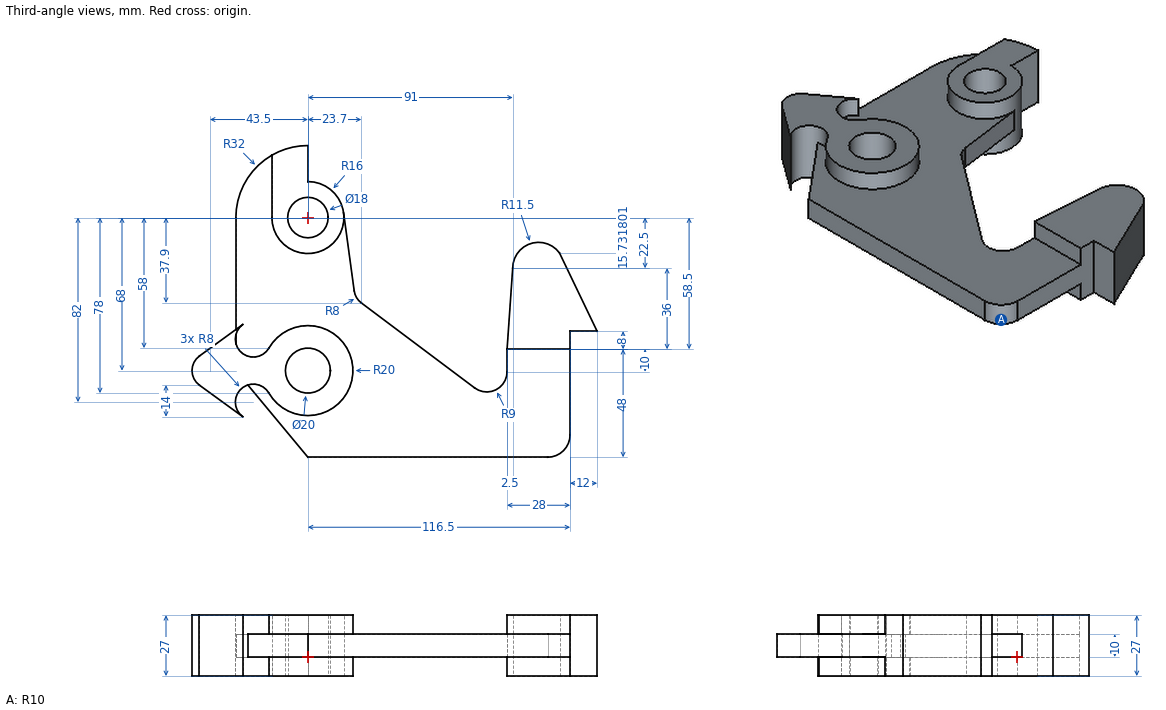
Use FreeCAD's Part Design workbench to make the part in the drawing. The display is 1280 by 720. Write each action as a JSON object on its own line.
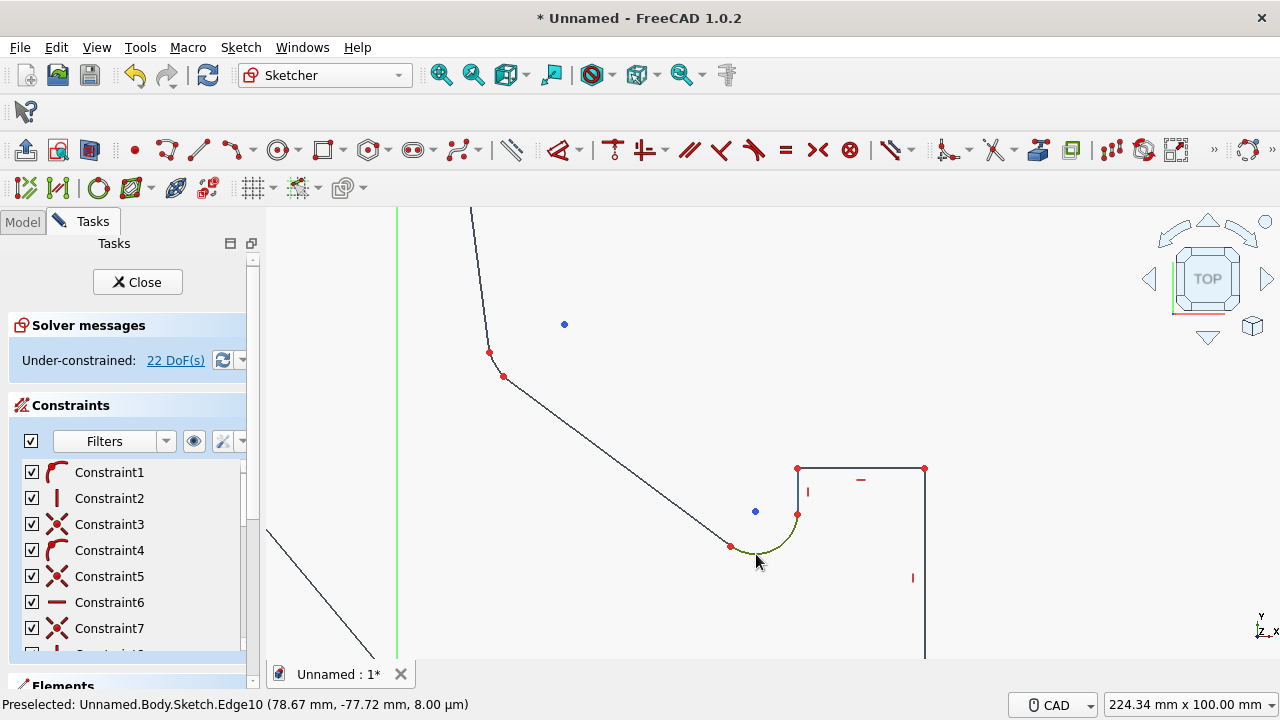
{"action": "left_click", "coordinate": [754, 150]}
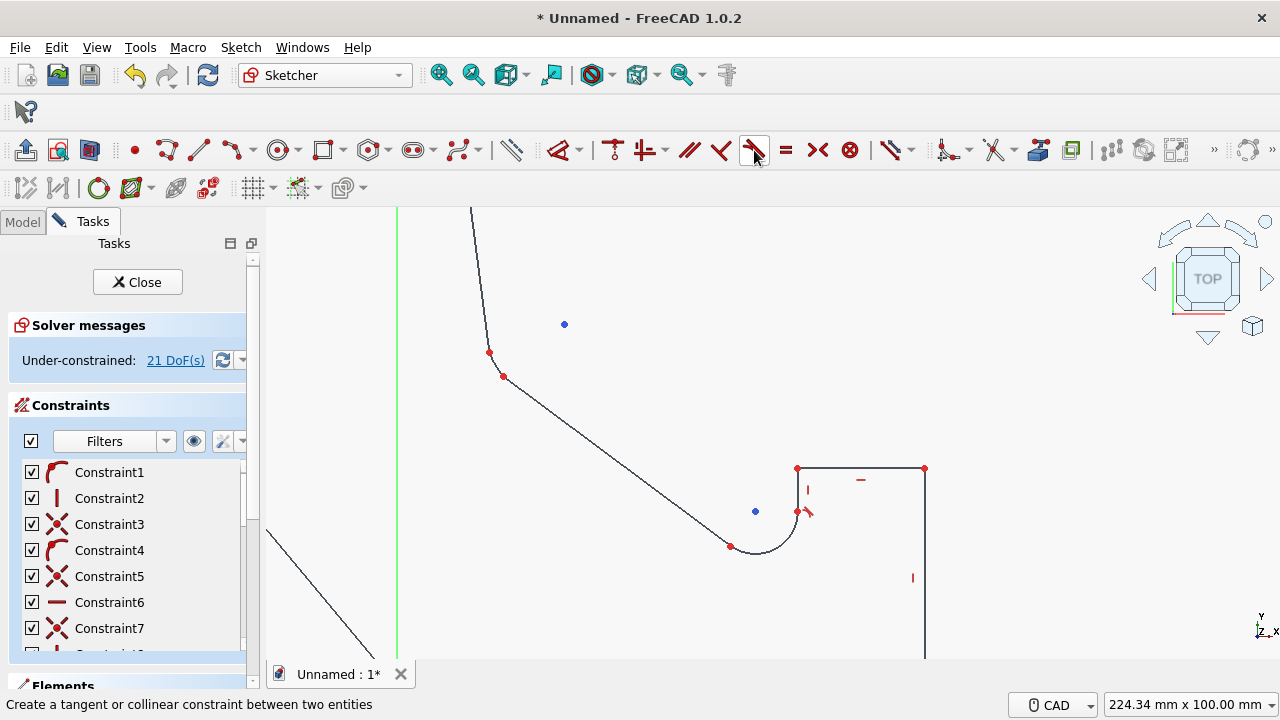
{"action": "left_click", "coordinate": [663, 495]}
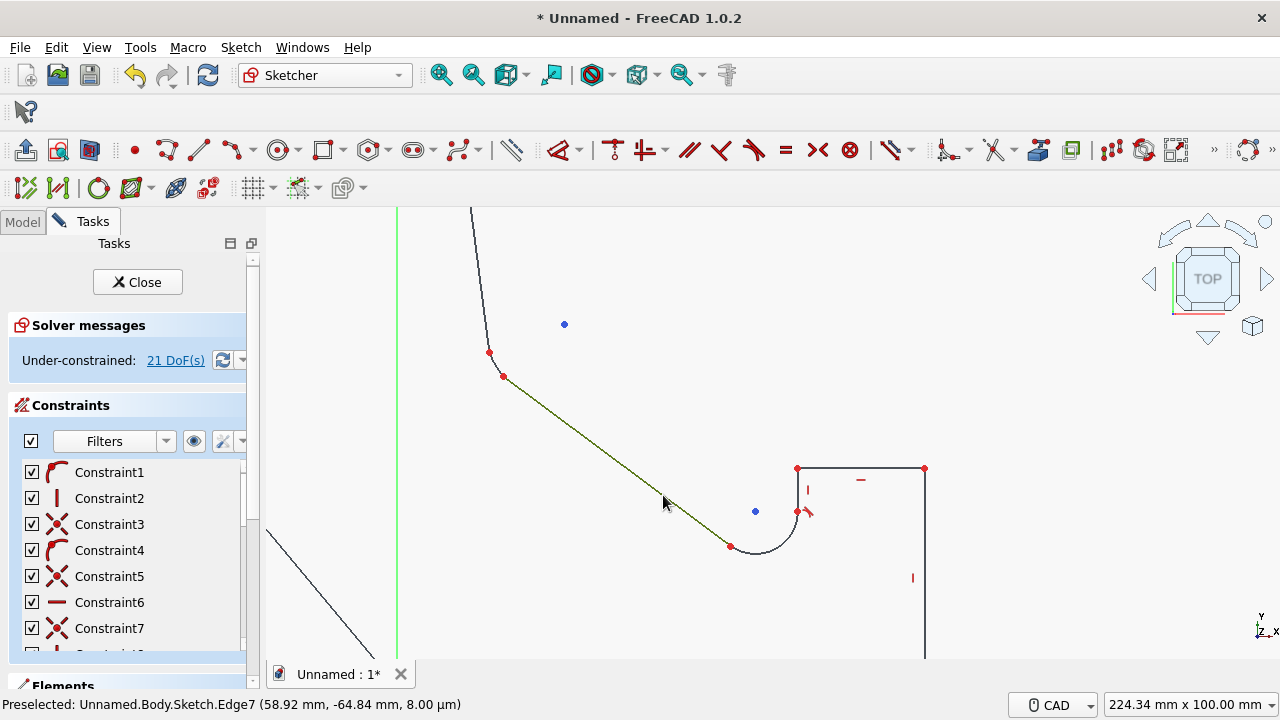
{"action": "left_click", "coordinate": [757, 554]}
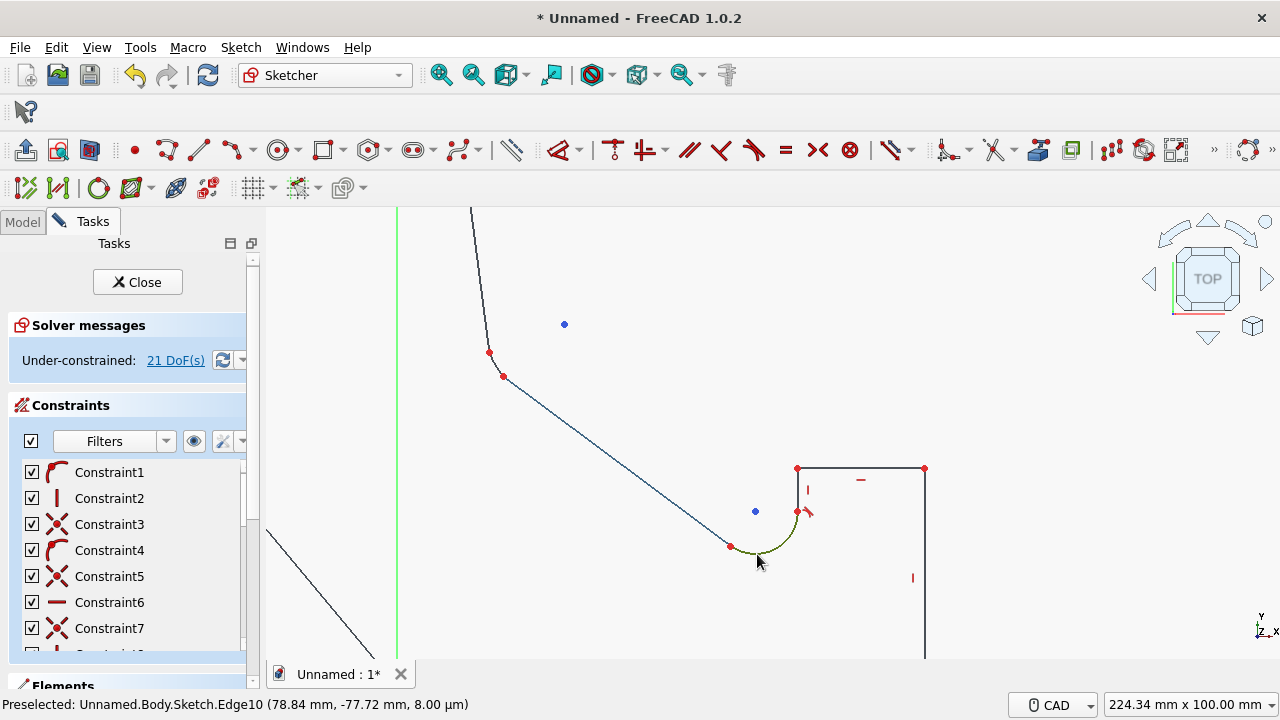
{"action": "left_click", "coordinate": [754, 150]}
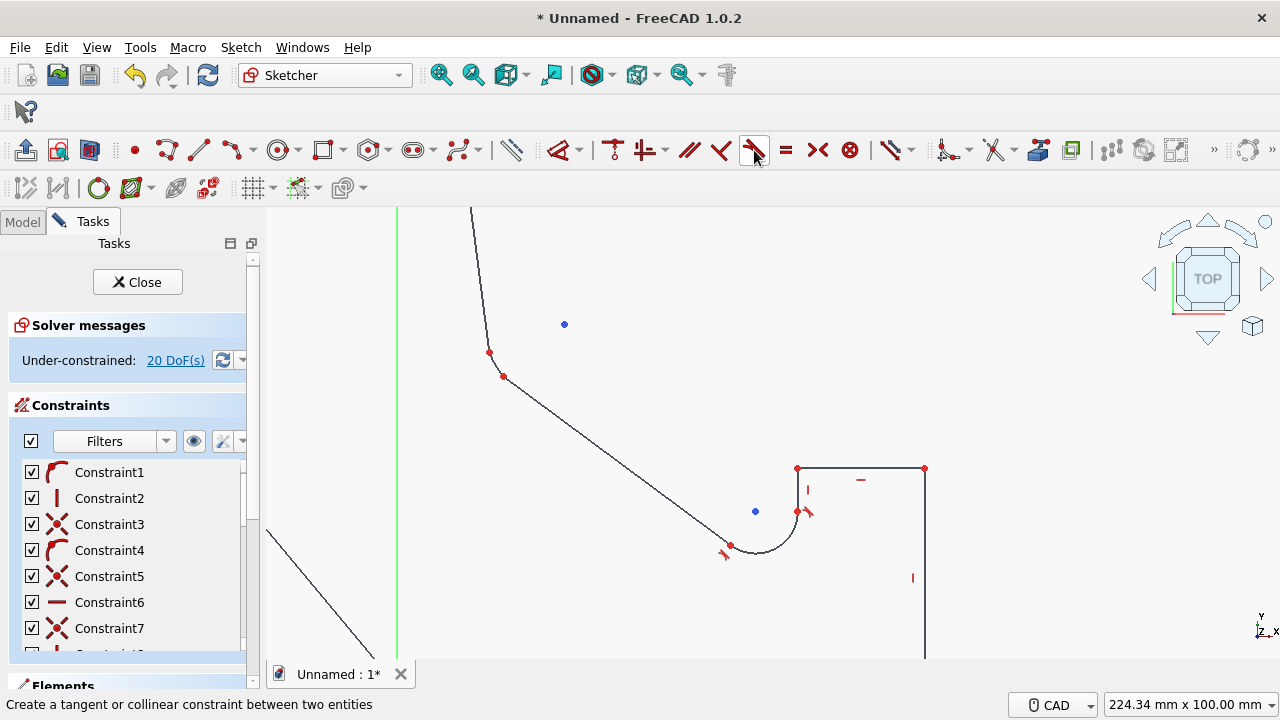
{"action": "left_click", "coordinate": [663, 495]}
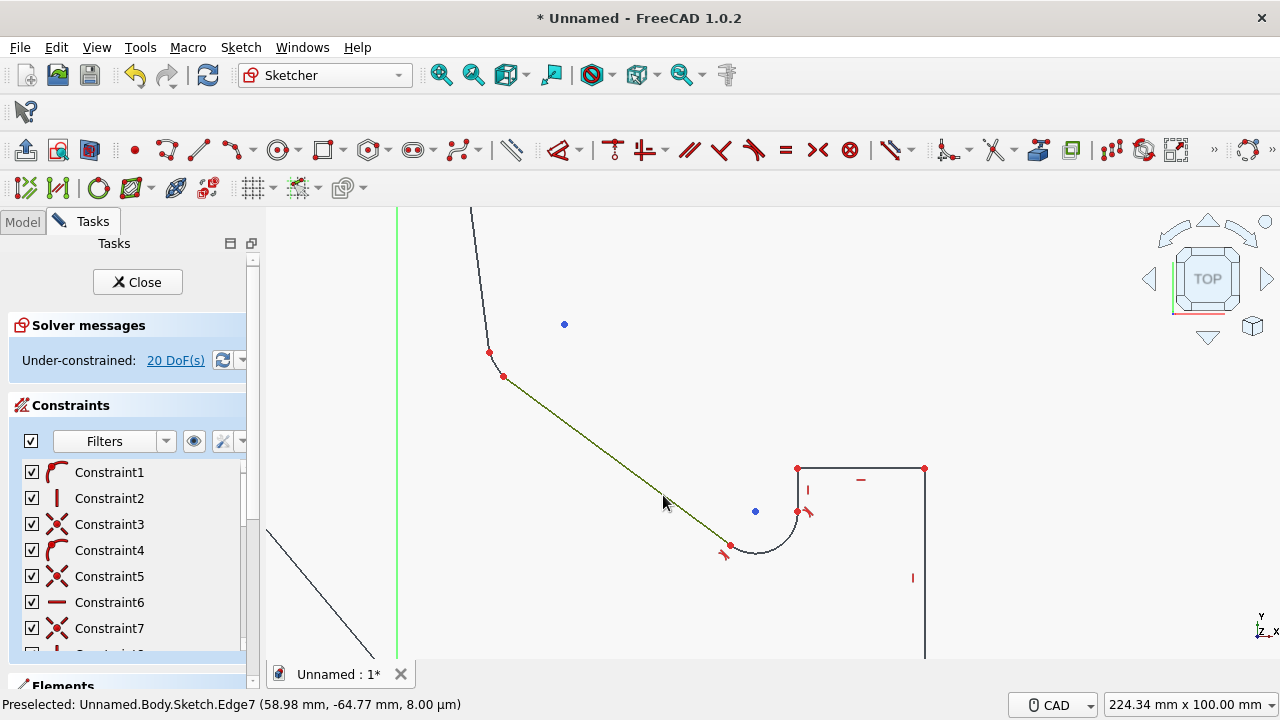
{"action": "left_click", "coordinate": [495, 365]}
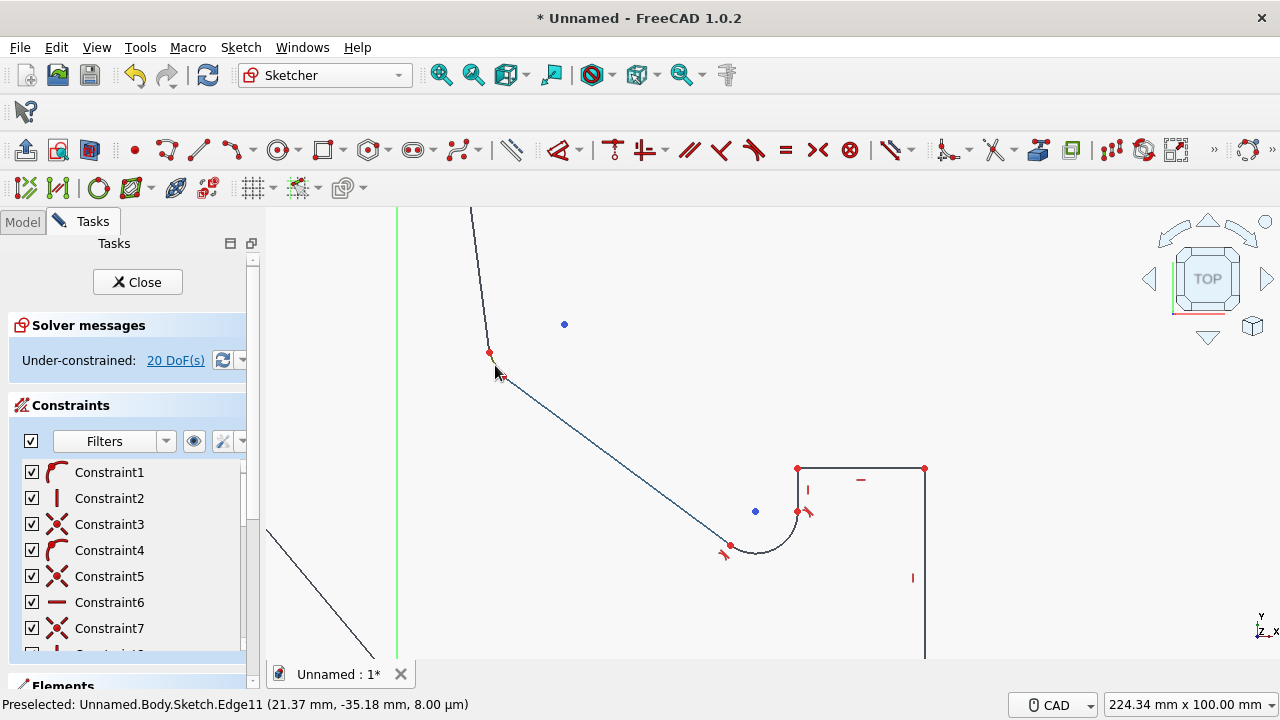
{"action": "left_click", "coordinate": [754, 150]}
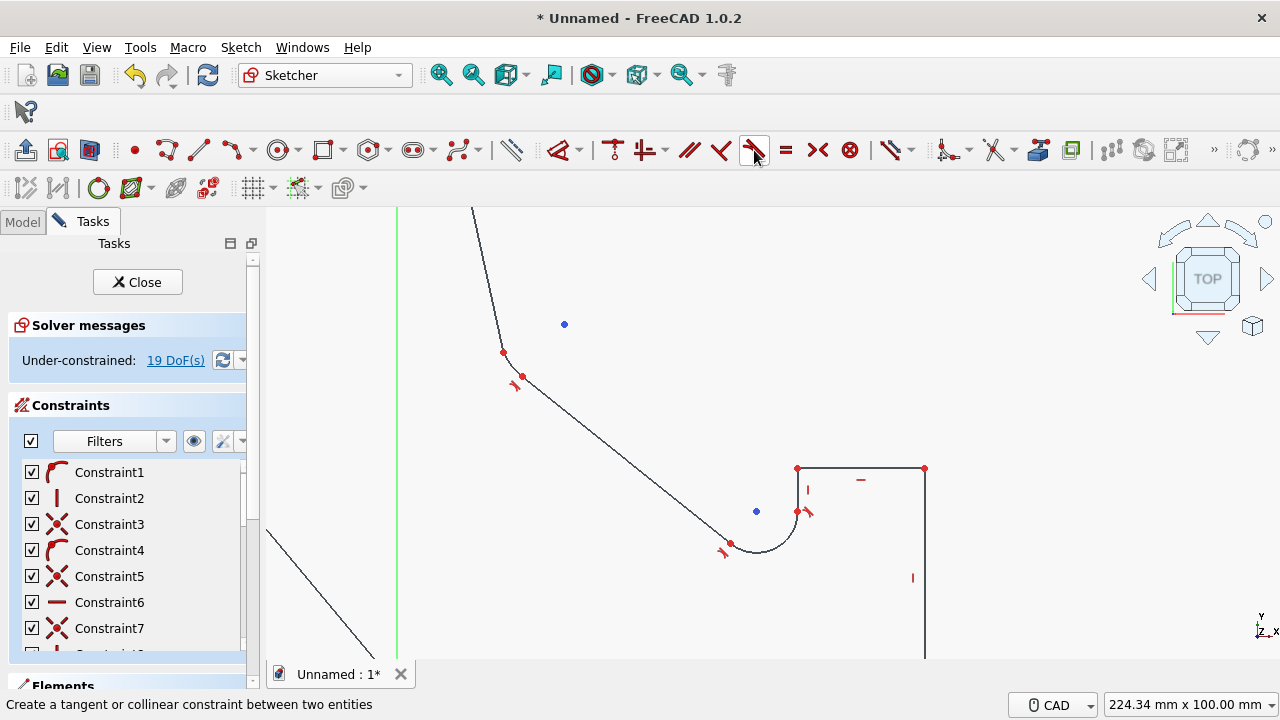
{"action": "left_click", "coordinate": [493, 304]}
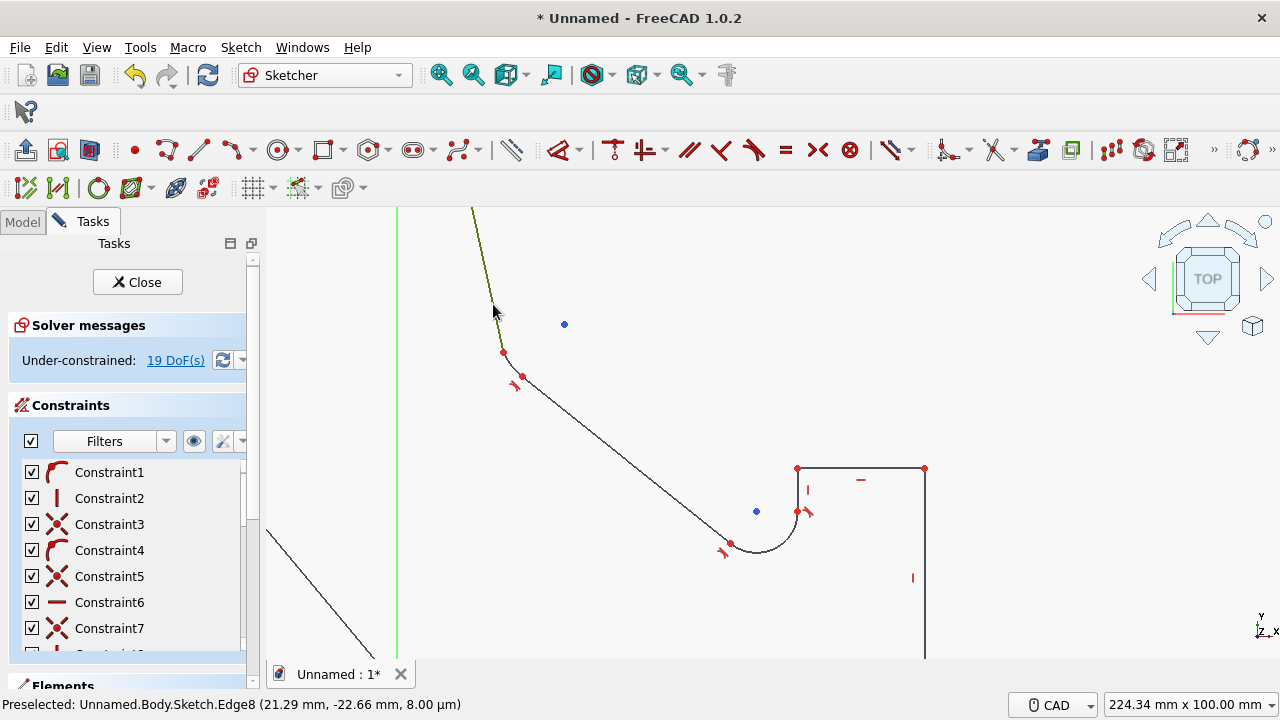
{"action": "scroll", "coordinate": [508, 360], "scroll_direction": "up", "scroll_amount": 2}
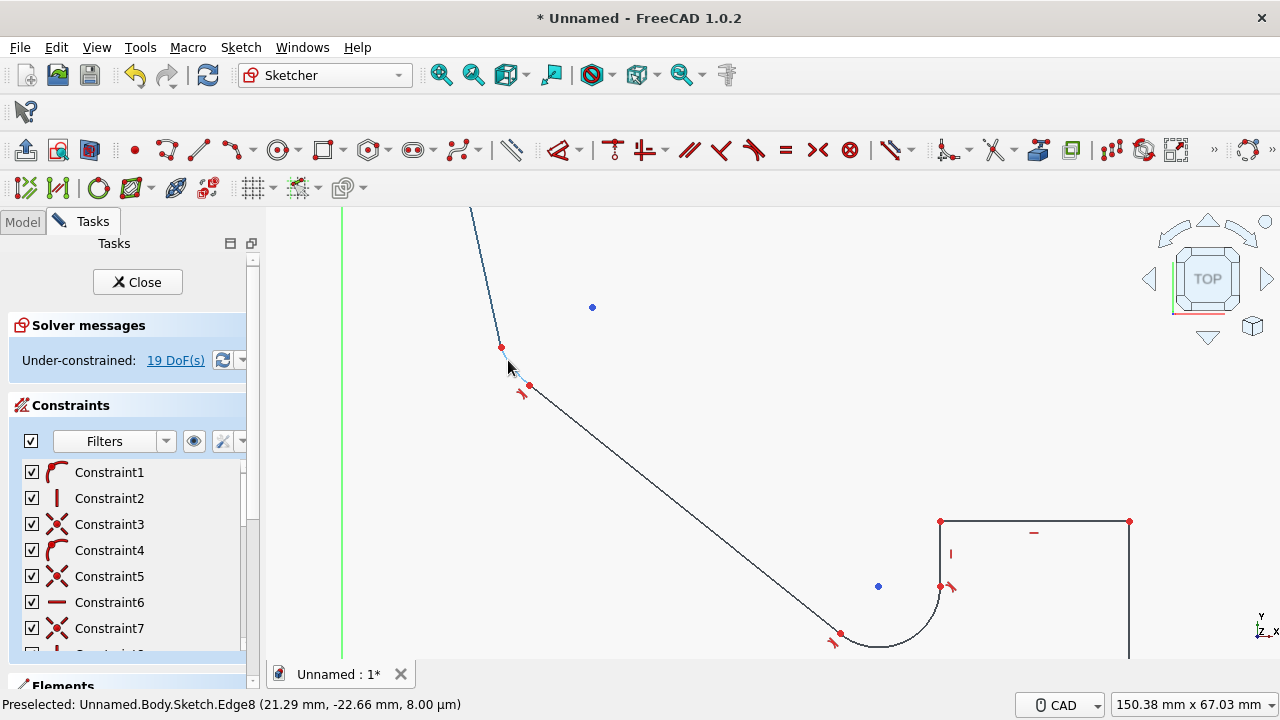
{"action": "left_click", "coordinate": [508, 360]}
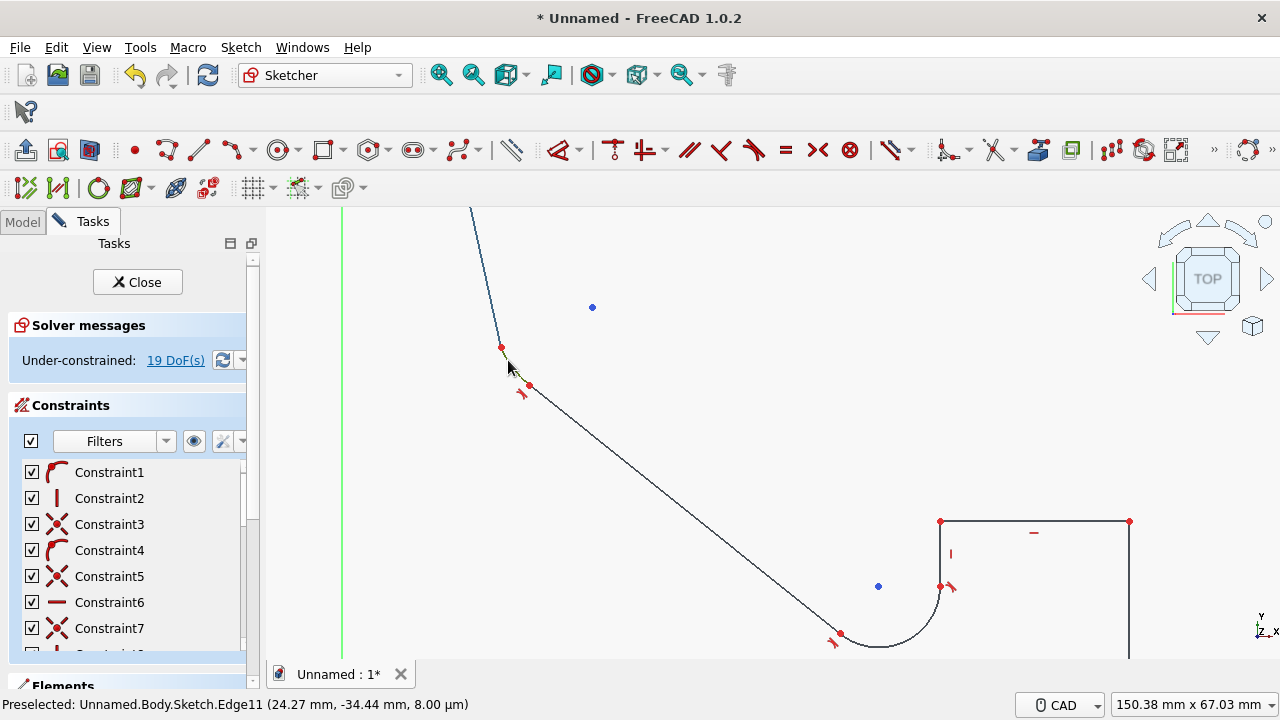
{"action": "left_click", "coordinate": [754, 150]}